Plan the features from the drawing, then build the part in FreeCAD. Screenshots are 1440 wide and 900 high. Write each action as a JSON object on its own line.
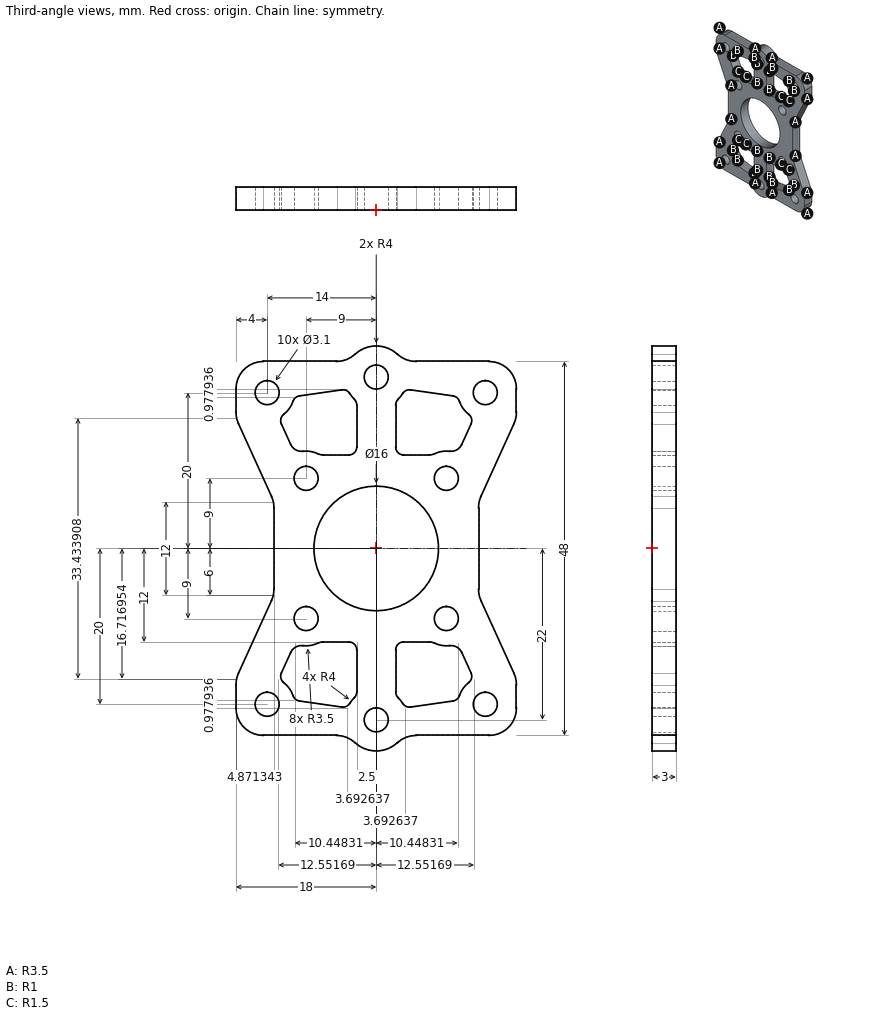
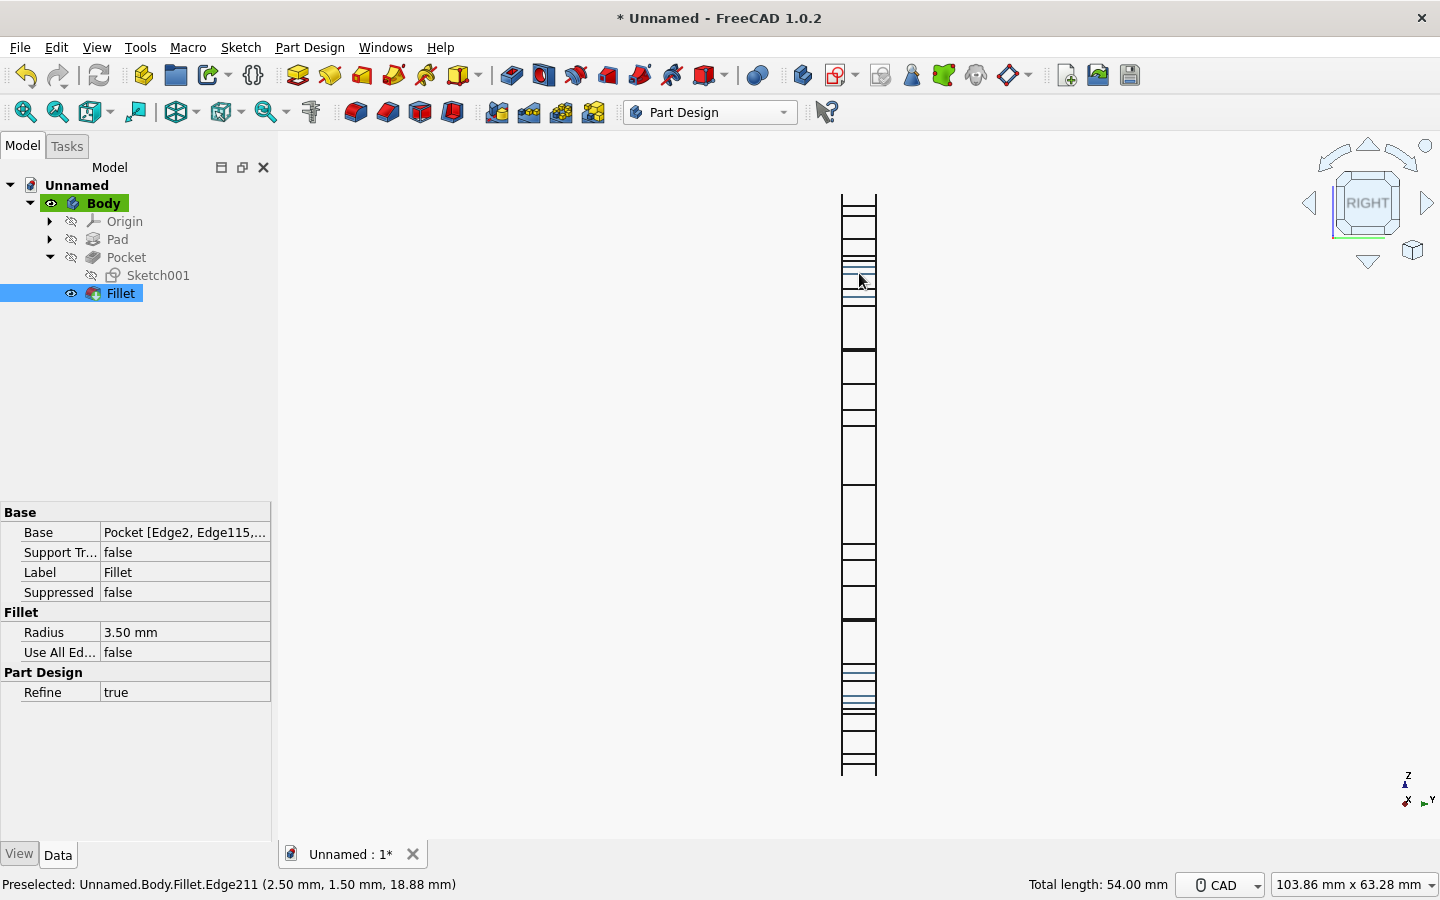
{"action": "key", "text": "5"}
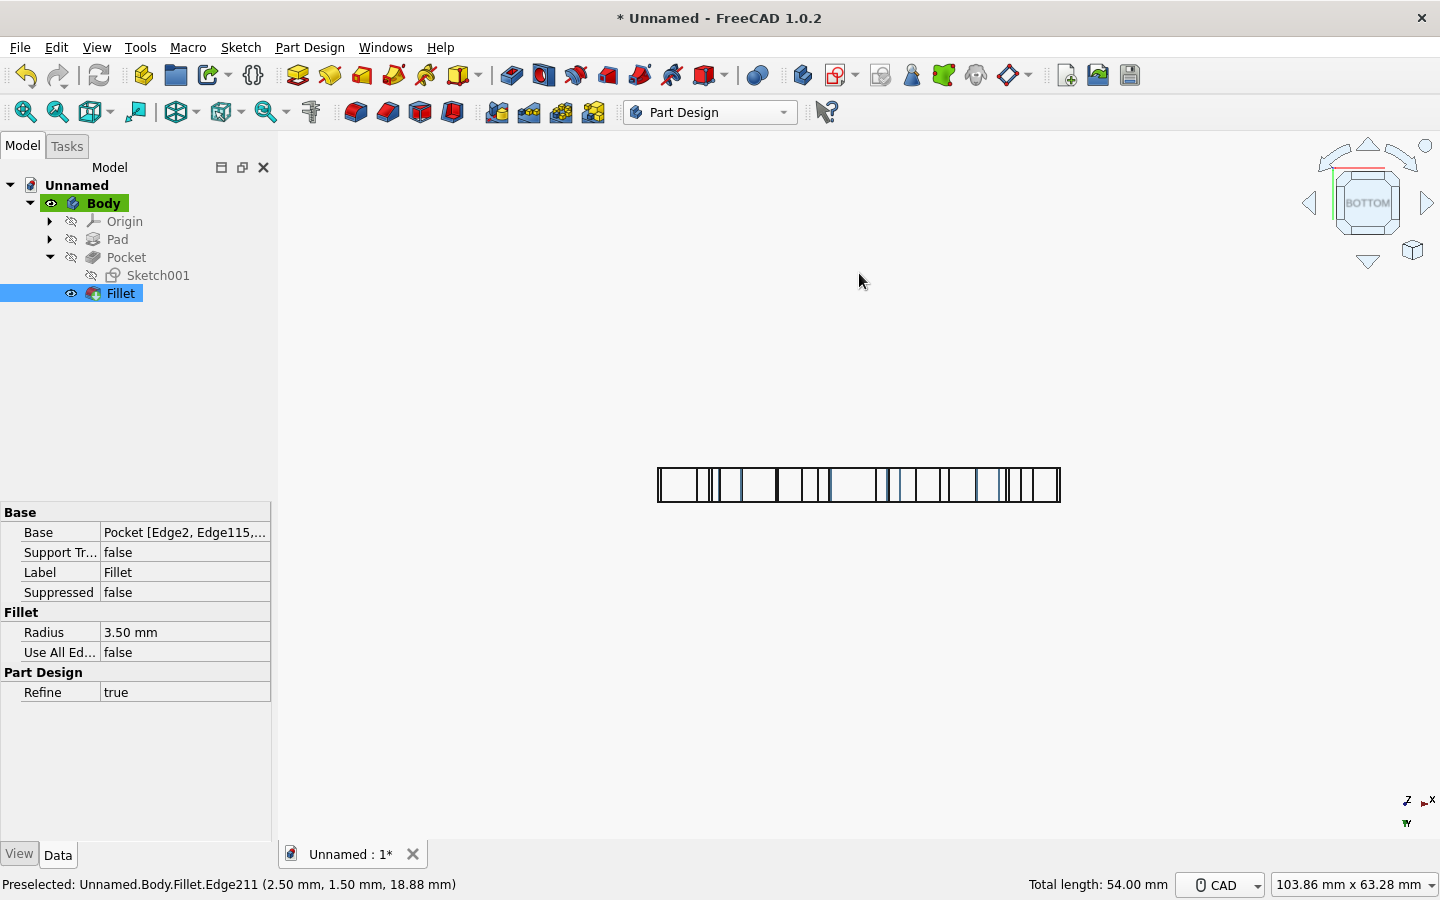
{"action": "key", "text": "v f"}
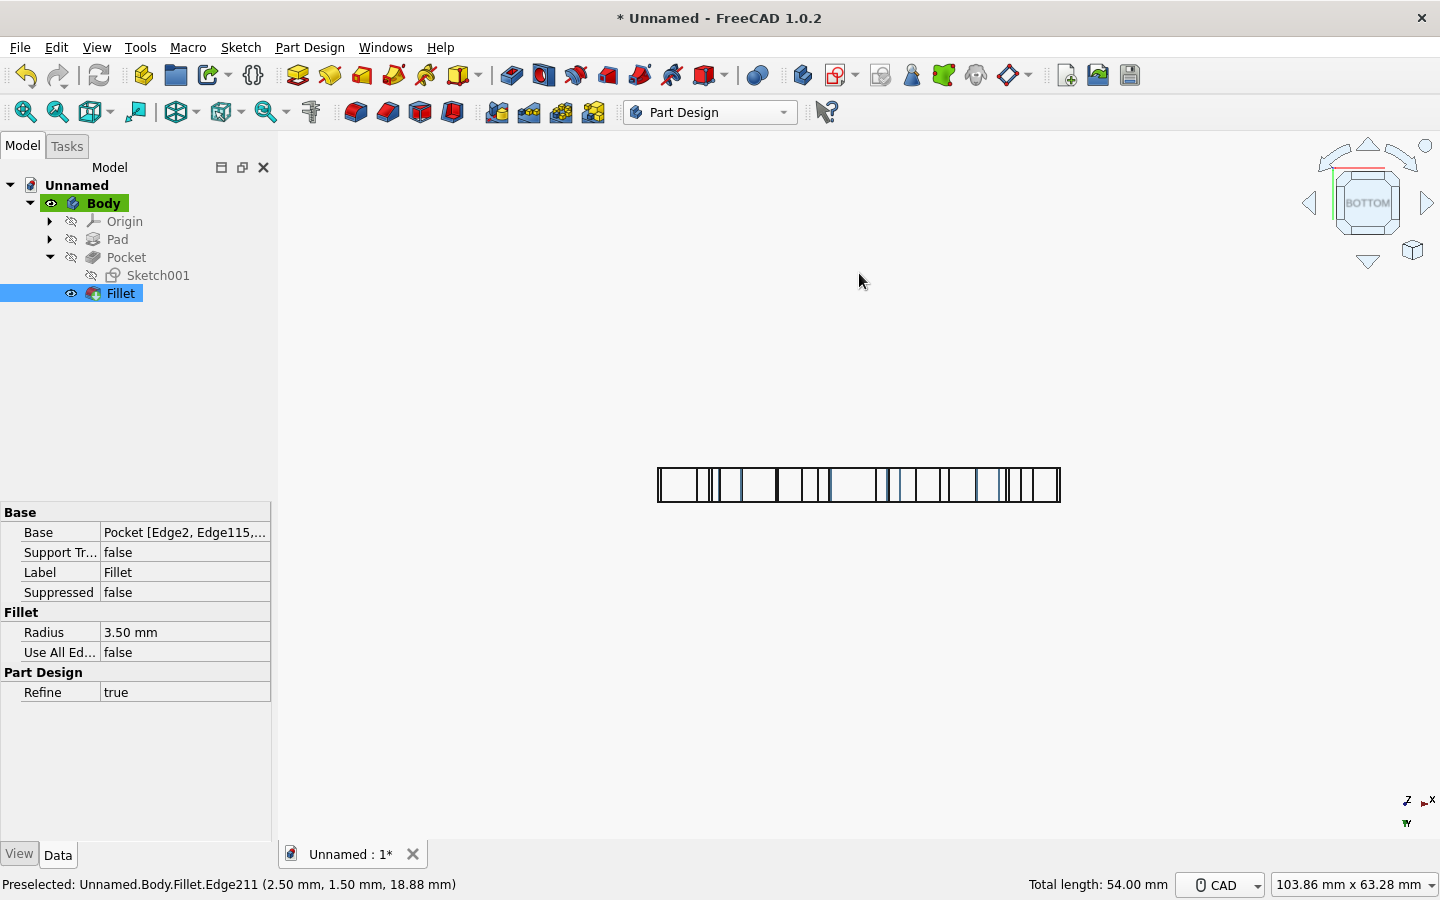
{"action": "left_click", "coordinate": [818, 484], "text": "ctrl"}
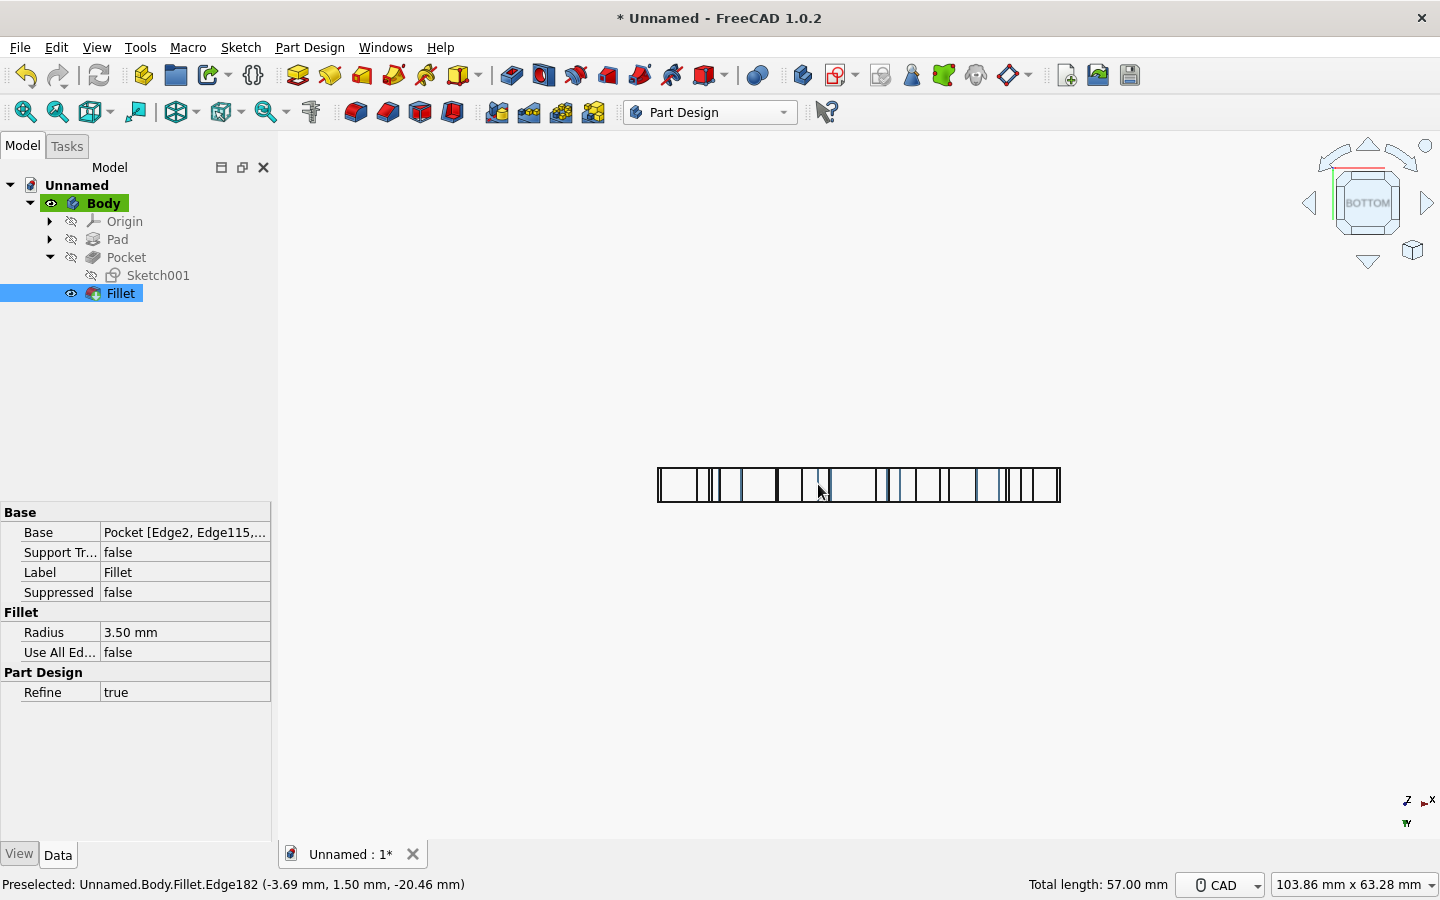
{"action": "key", "text": "4"}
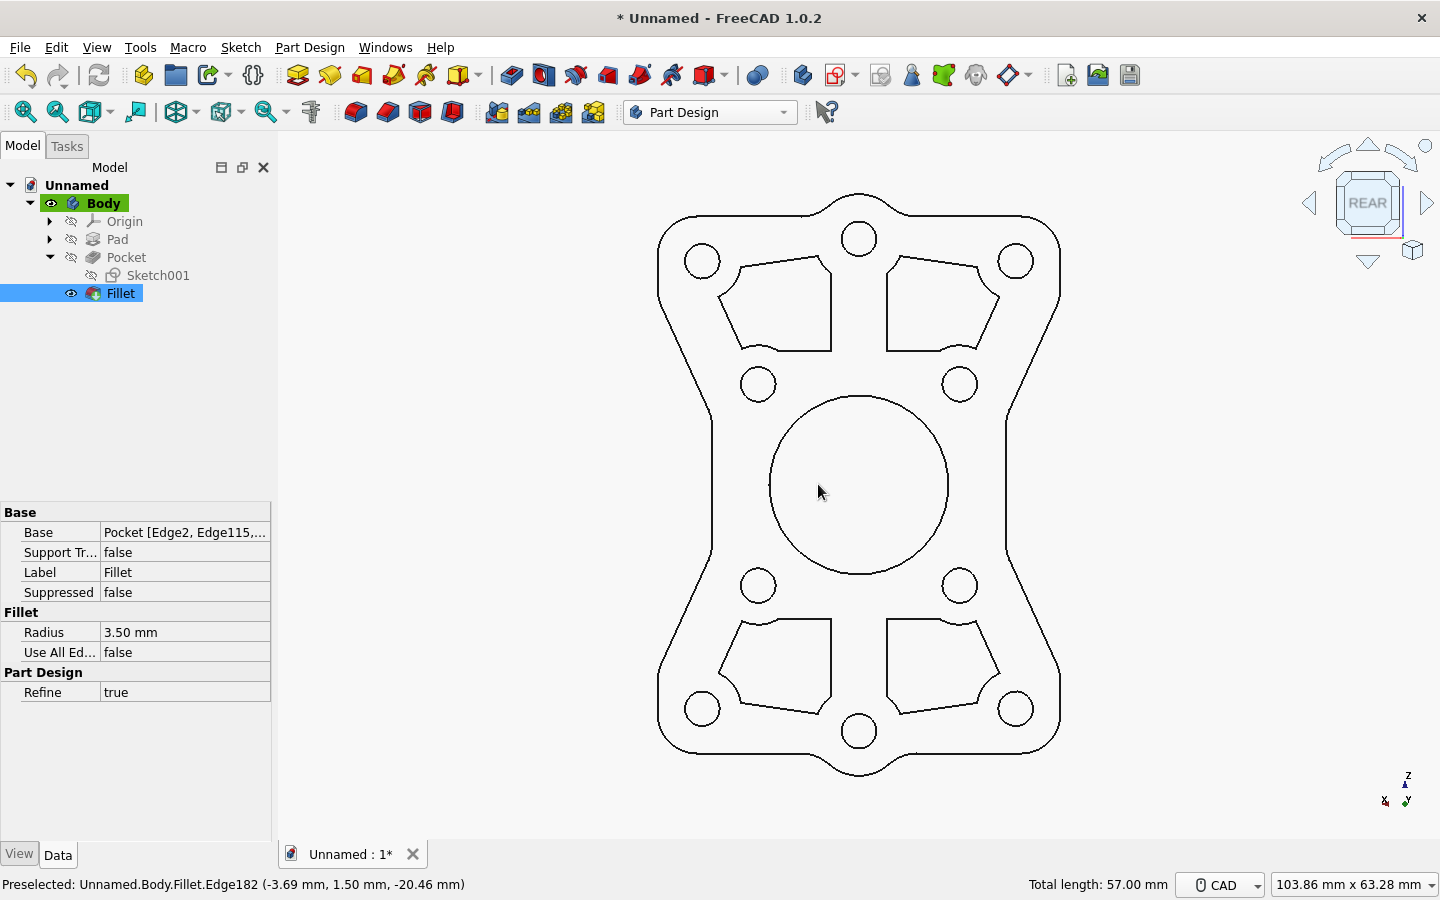
{"action": "key", "text": "6"}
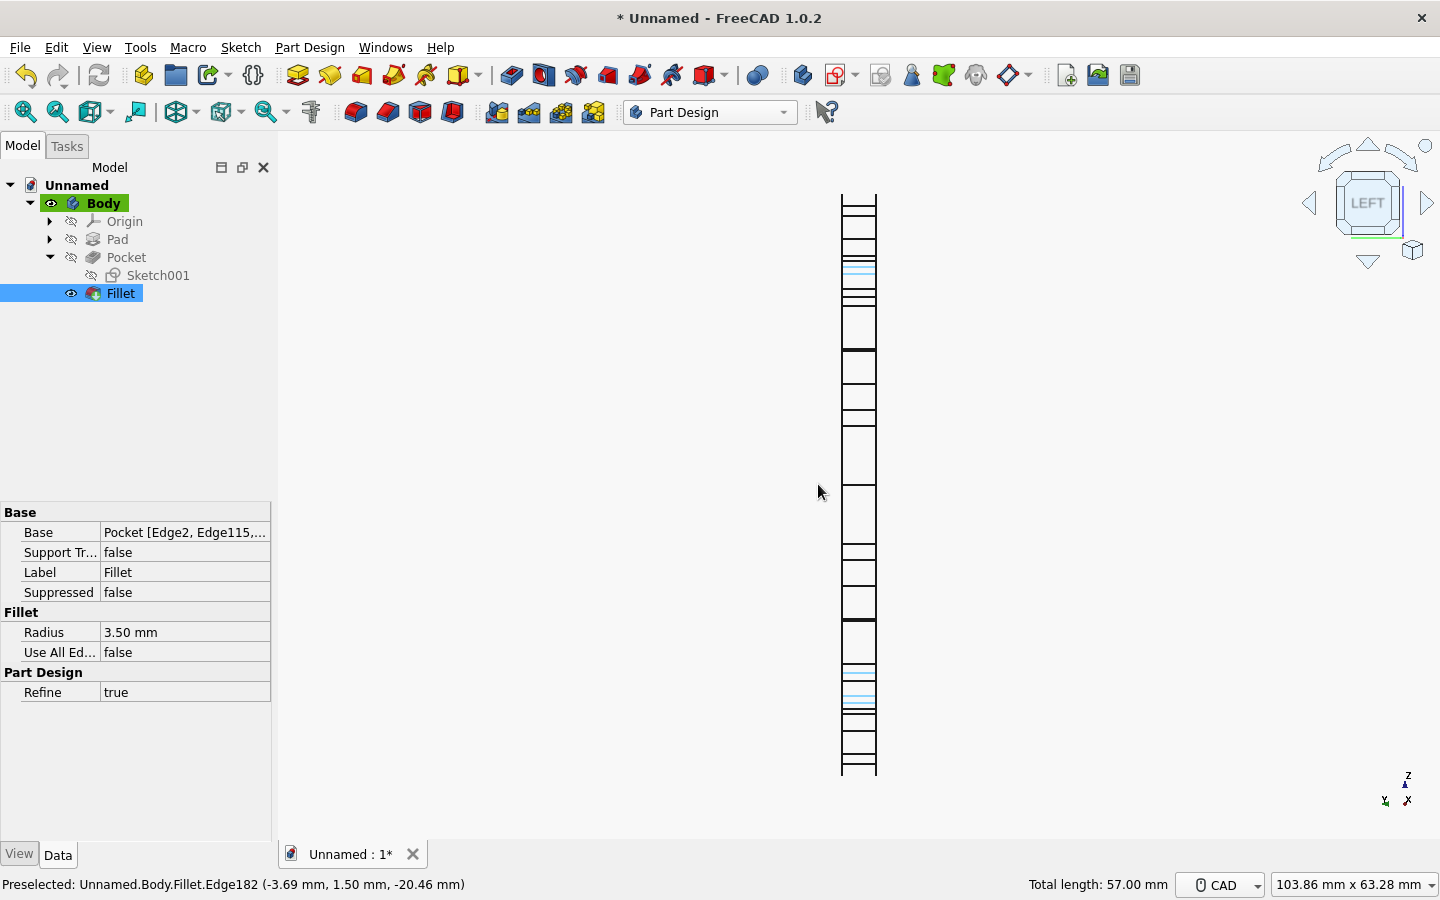
{"action": "left_click", "coordinate": [859, 296], "text": "ctrl"}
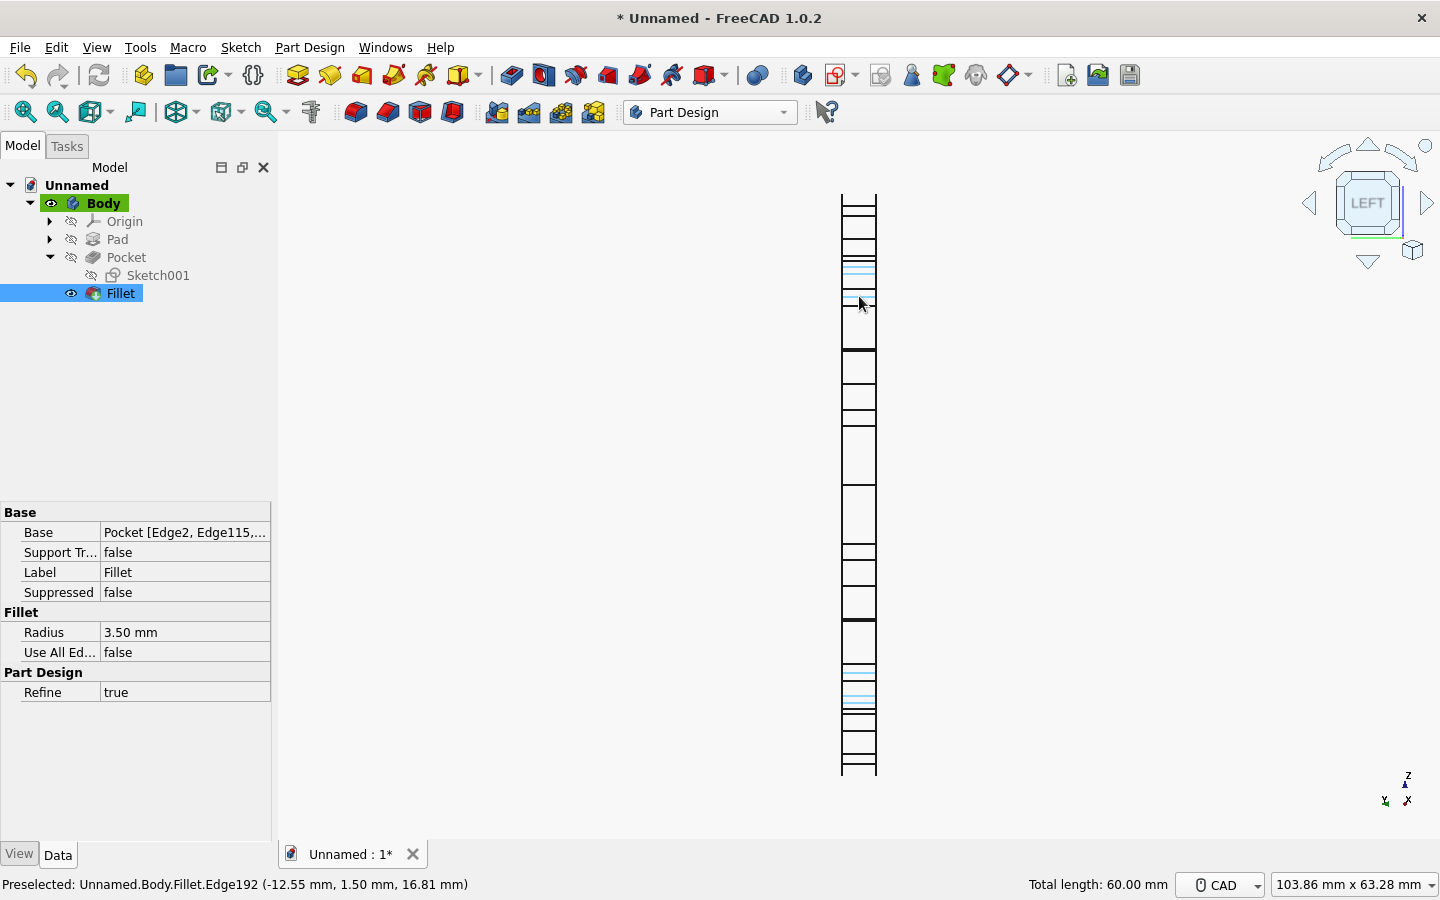
{"action": "key", "text": "v 1"}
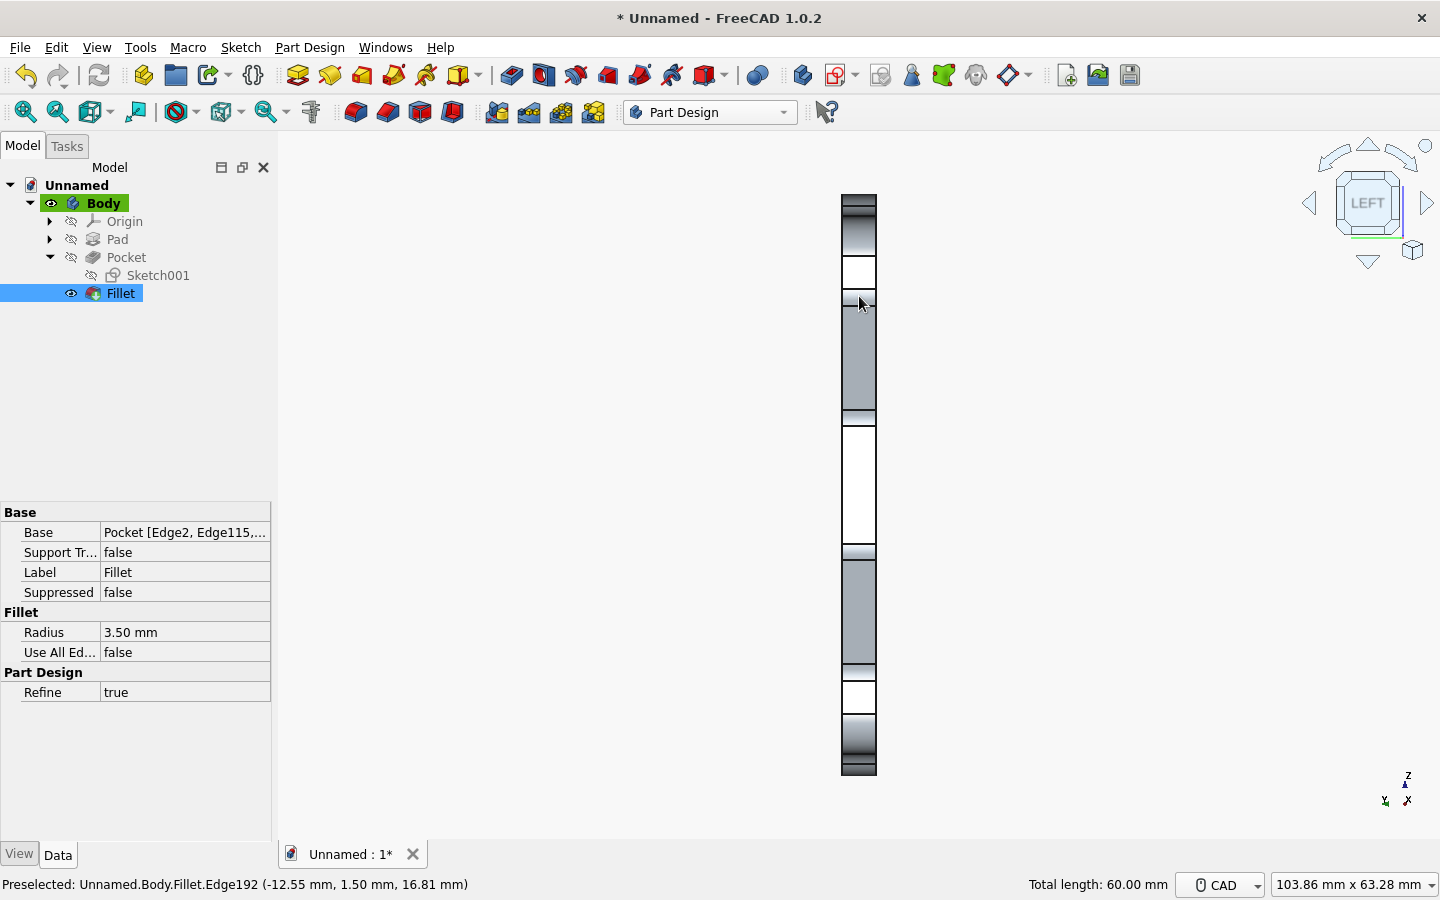
{"action": "left_click", "coordinate": [356, 112]}